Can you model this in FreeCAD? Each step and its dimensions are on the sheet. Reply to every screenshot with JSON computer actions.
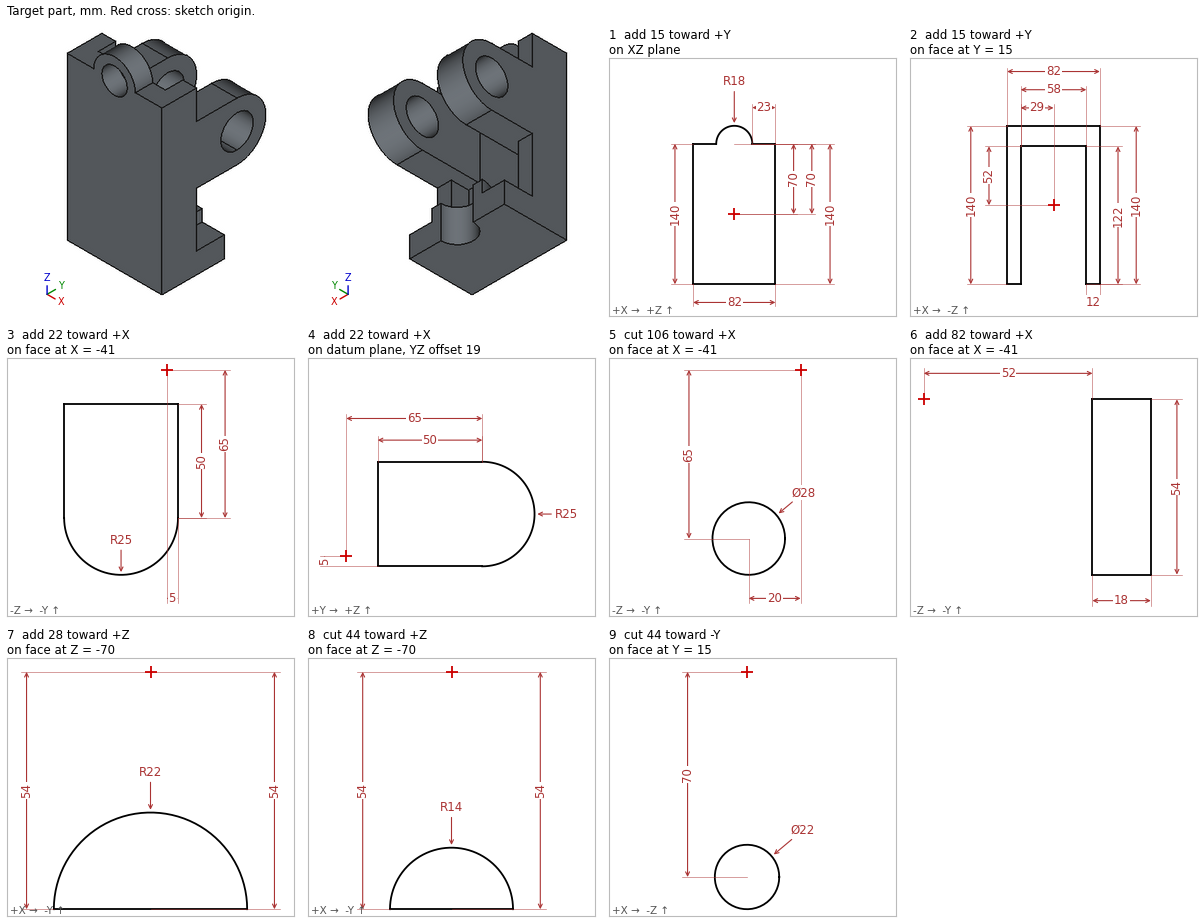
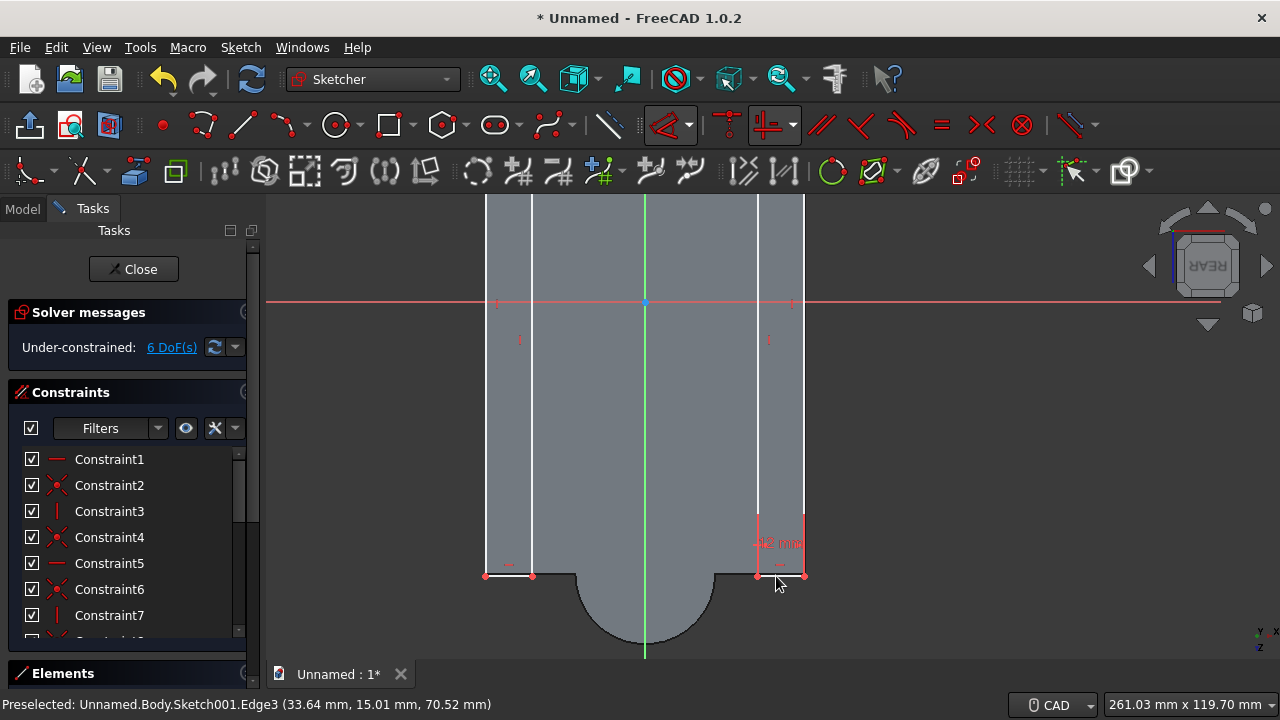
{"action": "scroll", "coordinate": [776, 577], "scroll_direction": "down", "scroll_amount": 3}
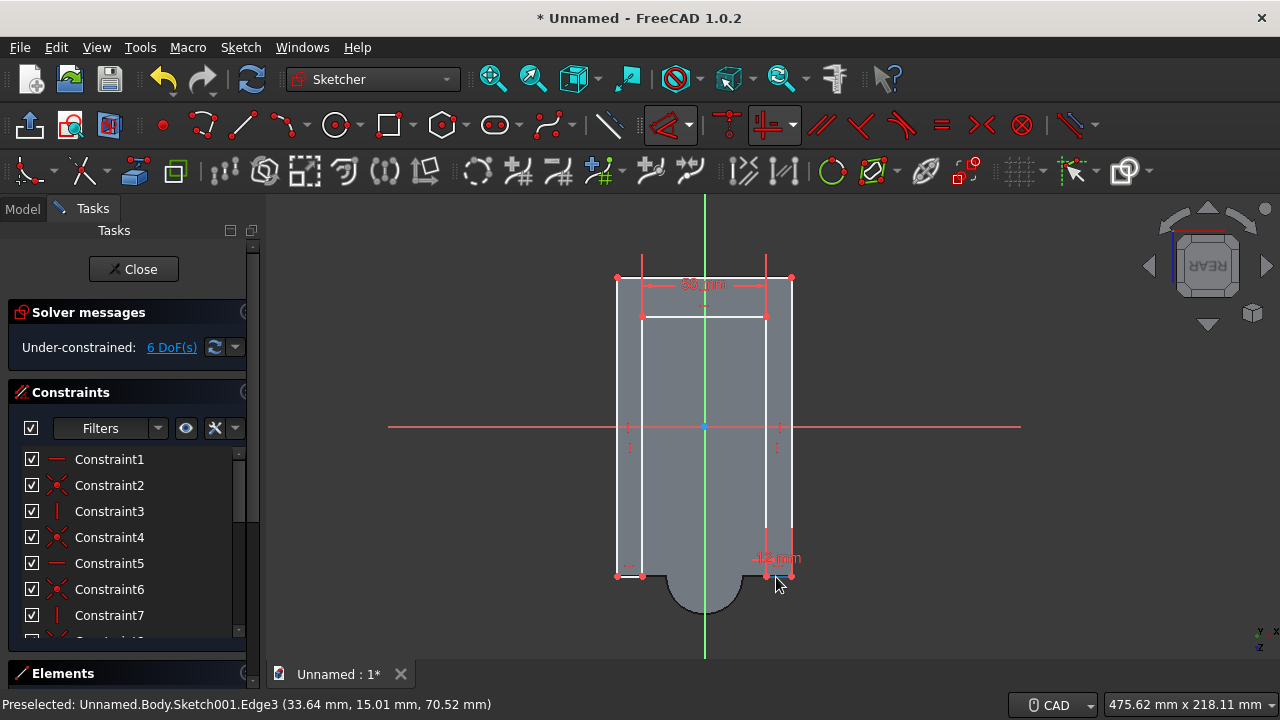
{"action": "left_click", "coordinate": [739, 278]}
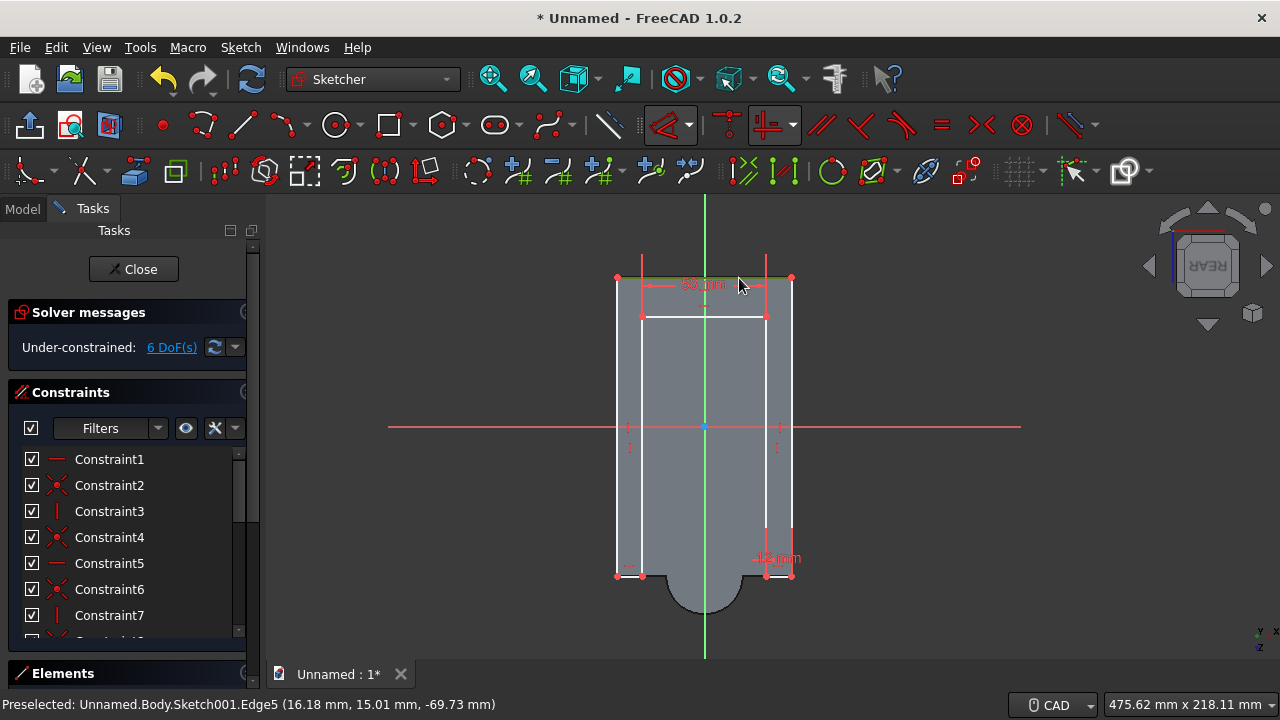
{"action": "key", "text": "l"}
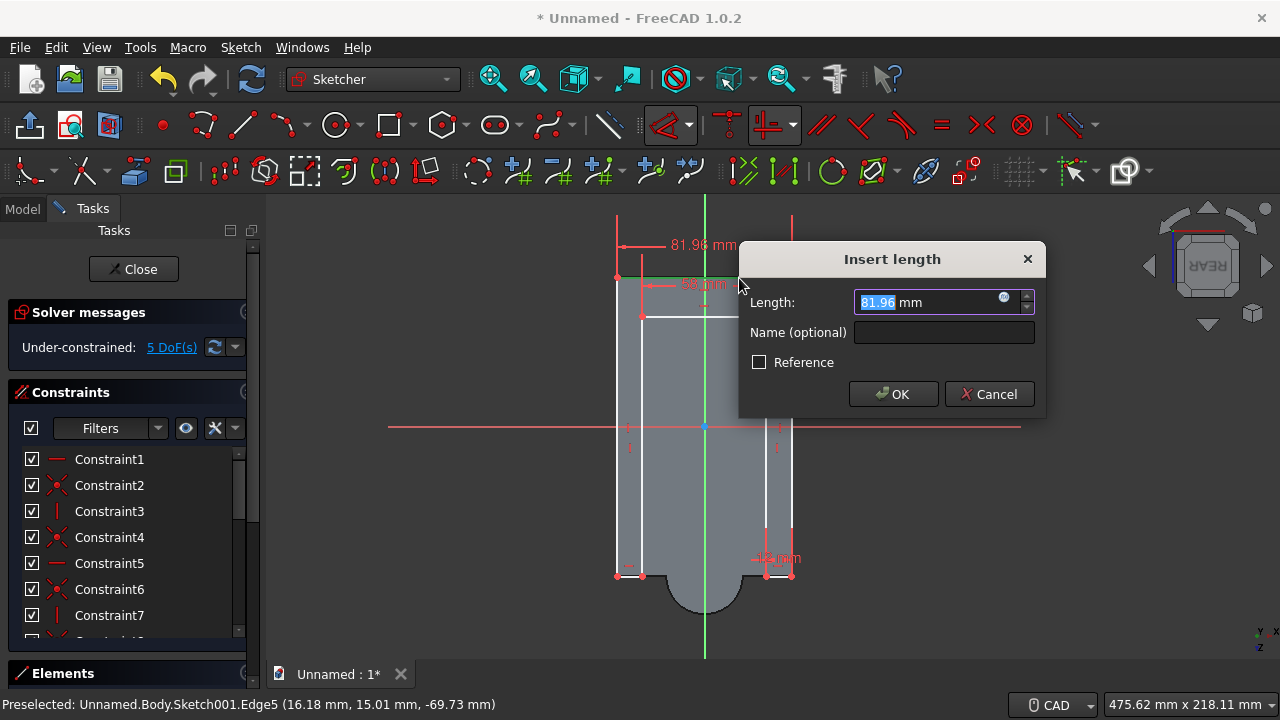
{"action": "type", "text": "82"}
{"action": "key", "text": "Return"}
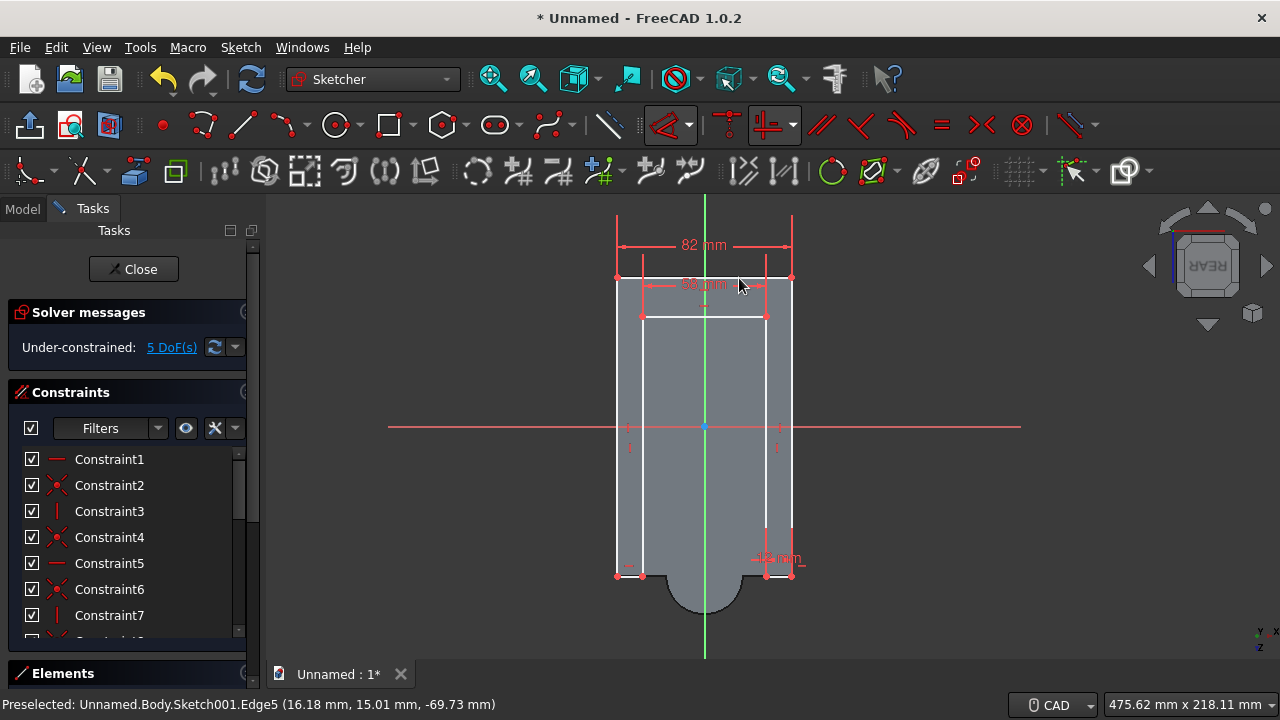
{"action": "left_click", "coordinate": [766, 395]}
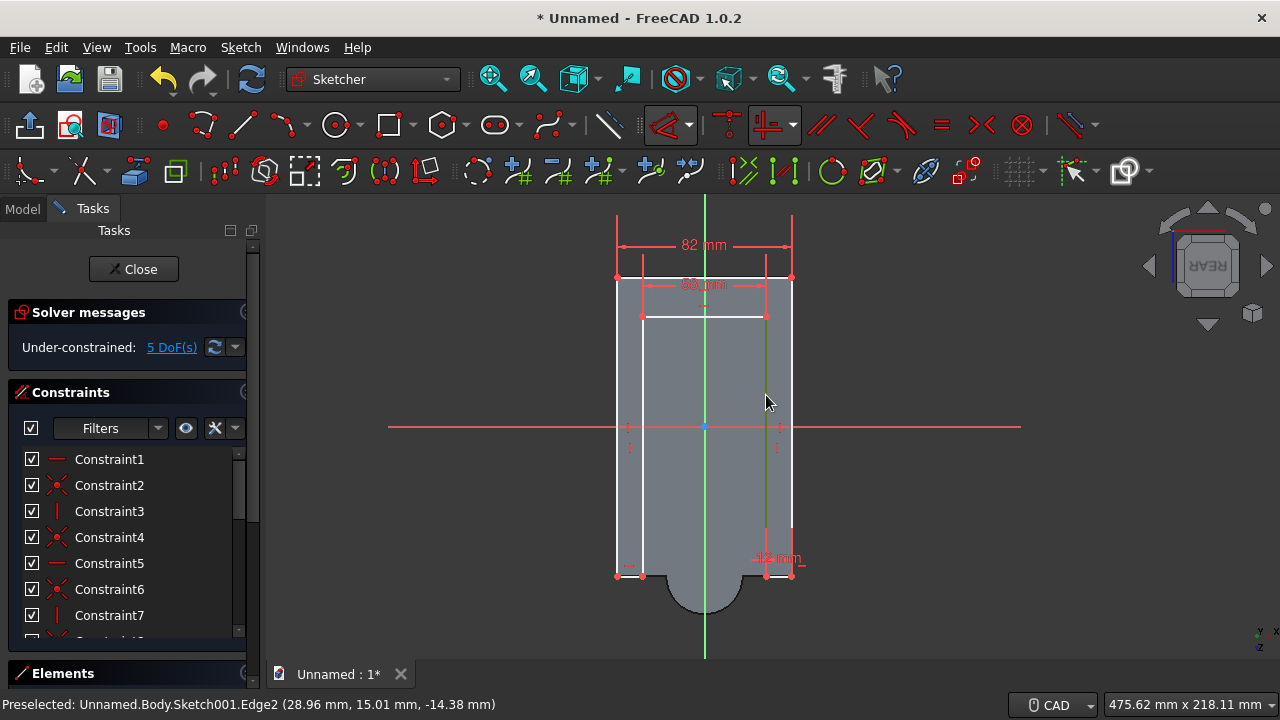
{"action": "key", "text": "i"}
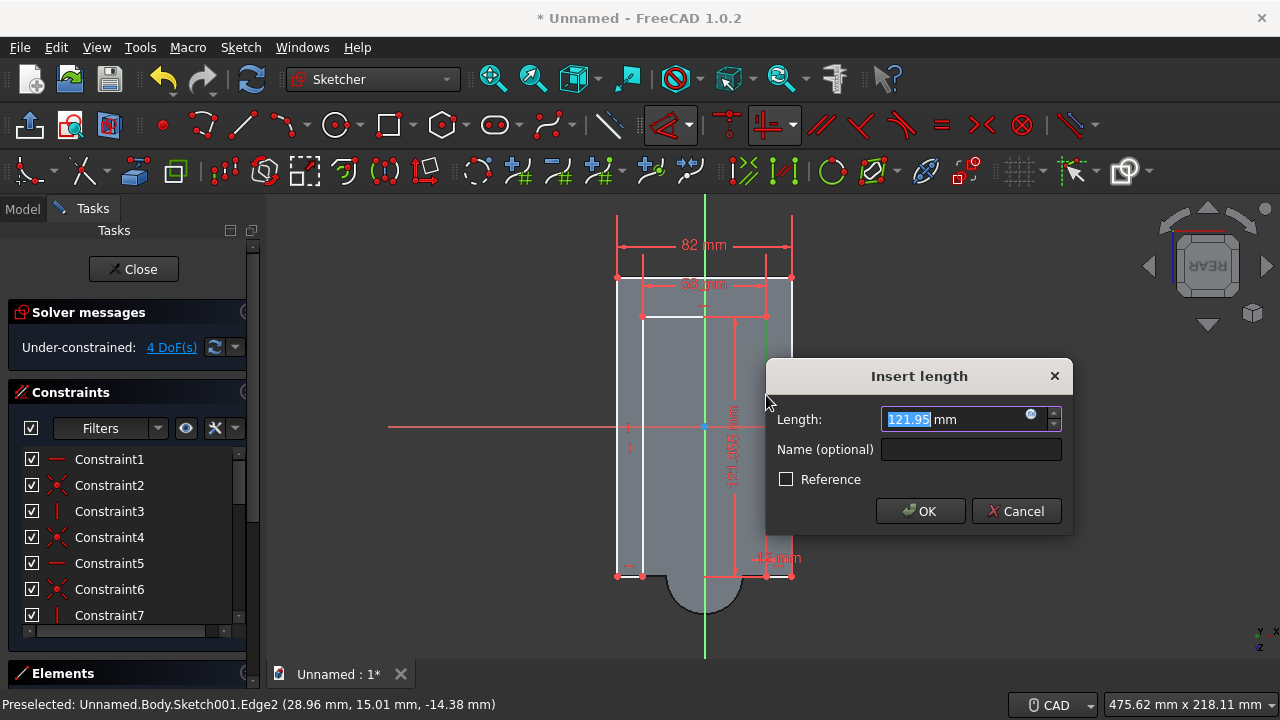
{"action": "type", "text": "122"}
{"action": "key", "text": "Return"}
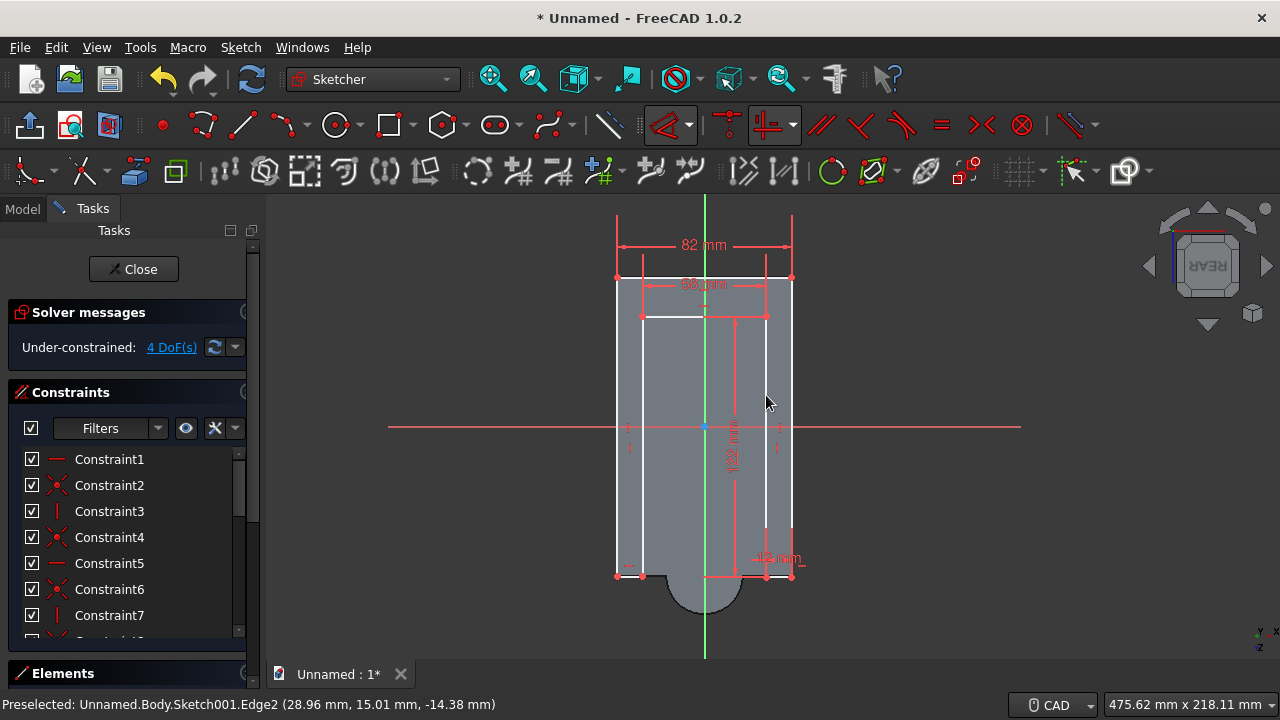
{"action": "left_click", "coordinate": [792, 487]}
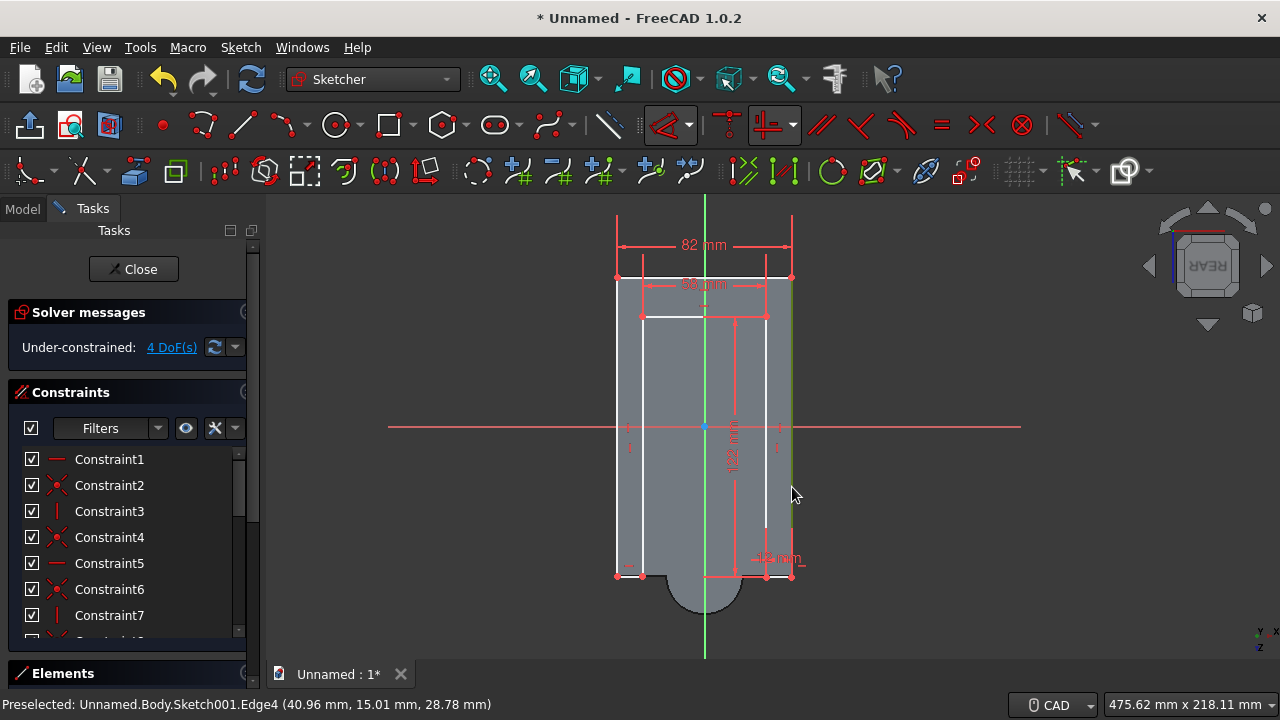
{"action": "key", "text": "i"}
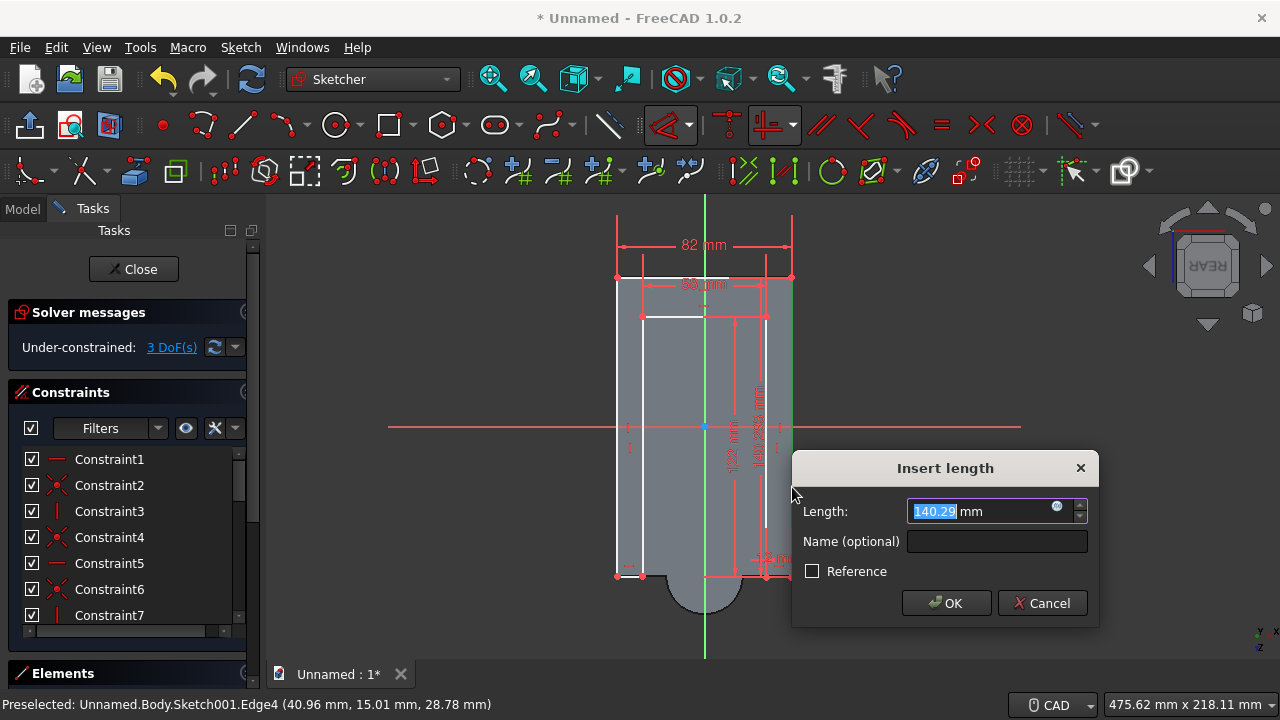
{"action": "type", "text": "140"}
{"action": "key", "text": "Return"}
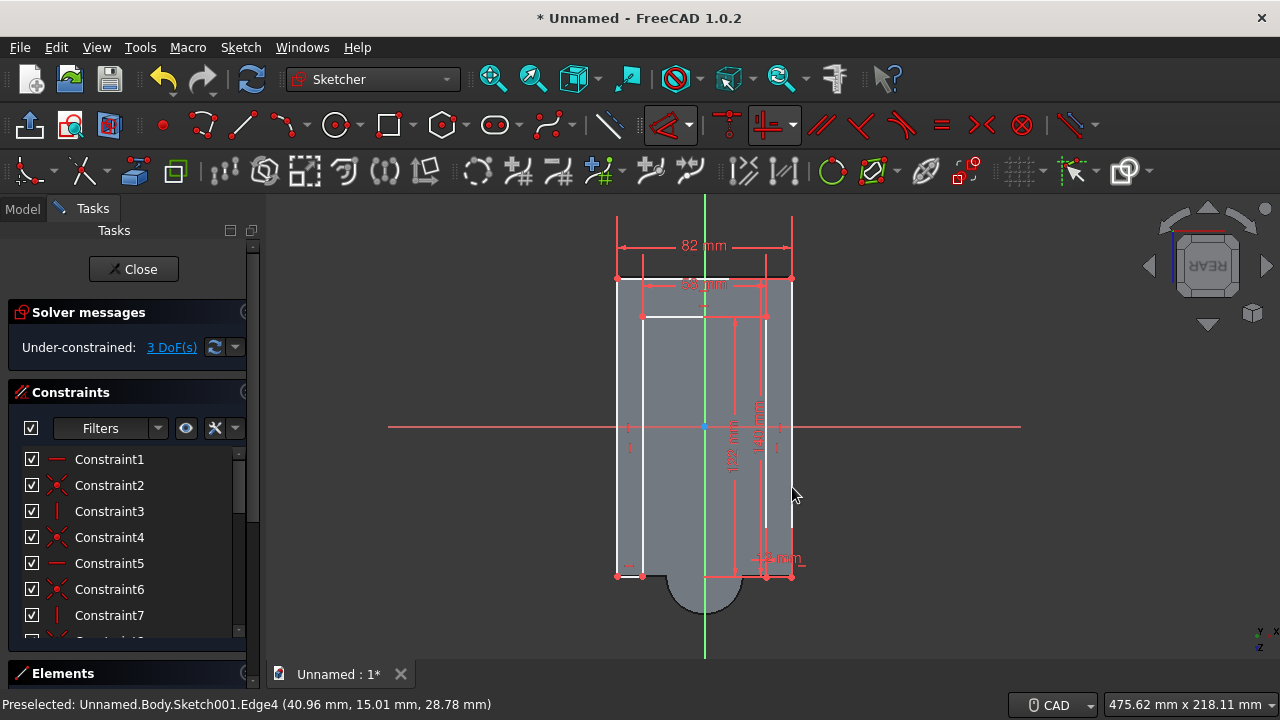
{"action": "left_click", "coordinate": [617, 368]}